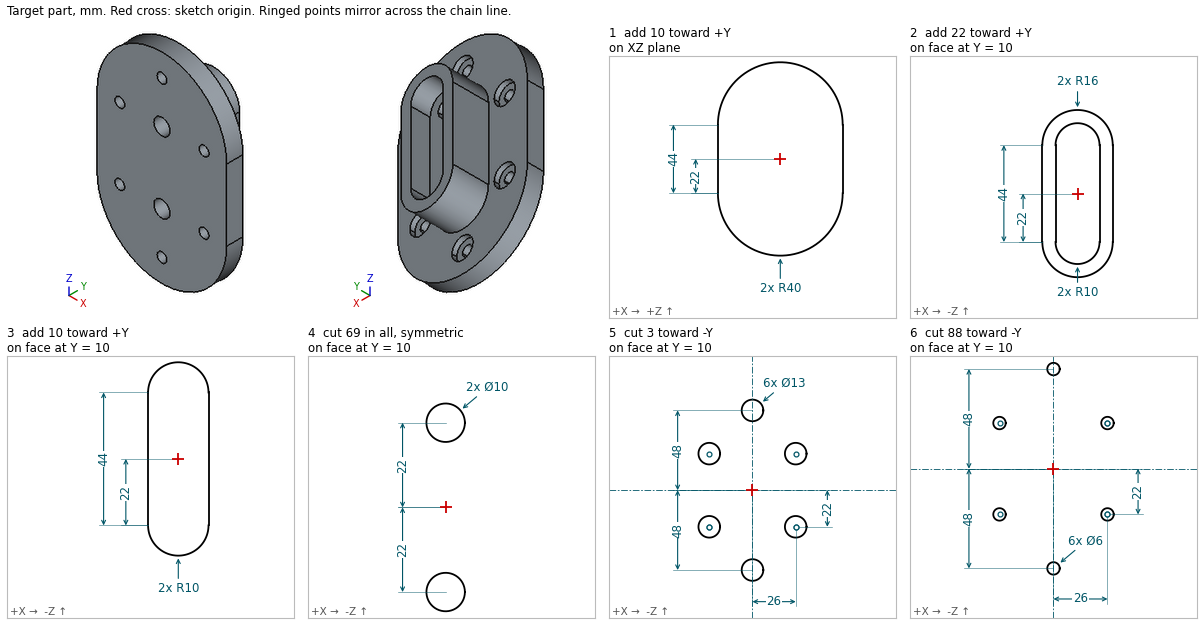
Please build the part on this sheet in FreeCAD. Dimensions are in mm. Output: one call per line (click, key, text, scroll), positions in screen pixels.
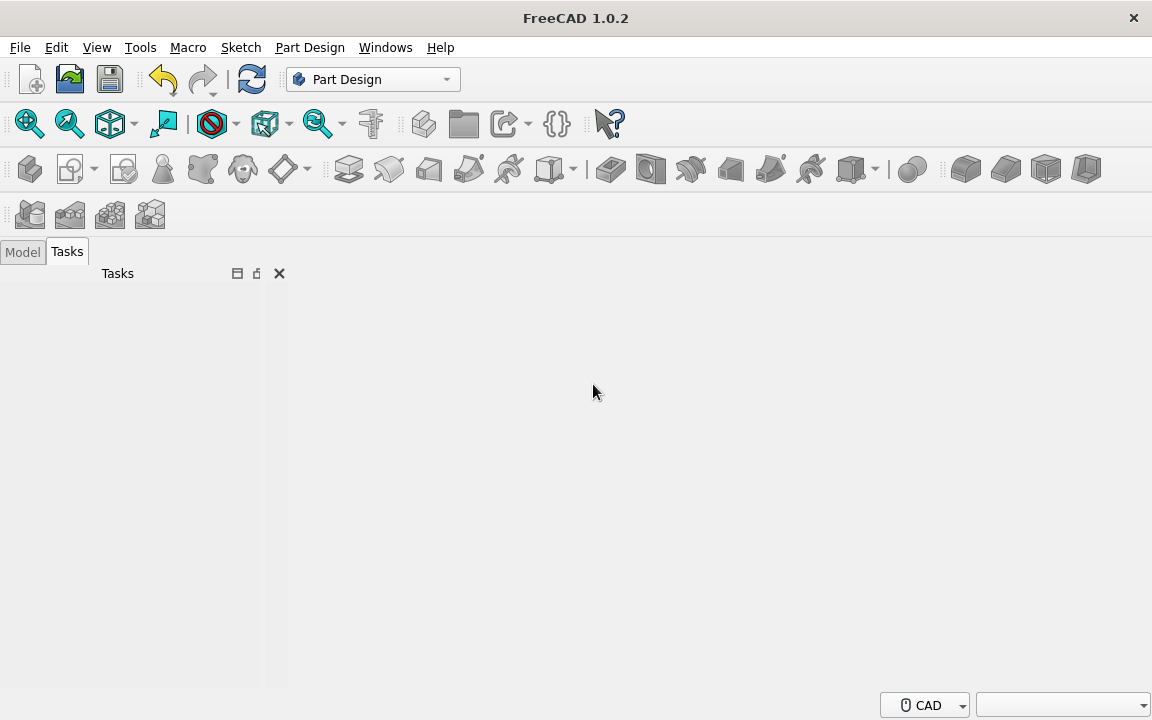
click(30, 80)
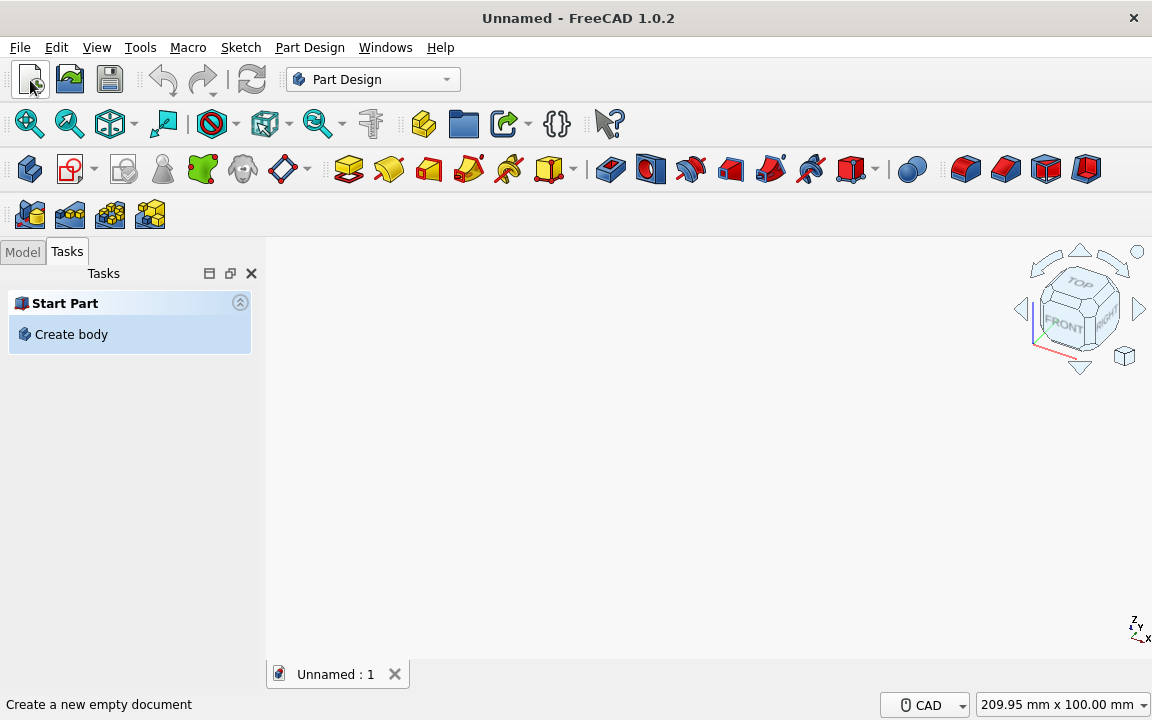
click(70, 170)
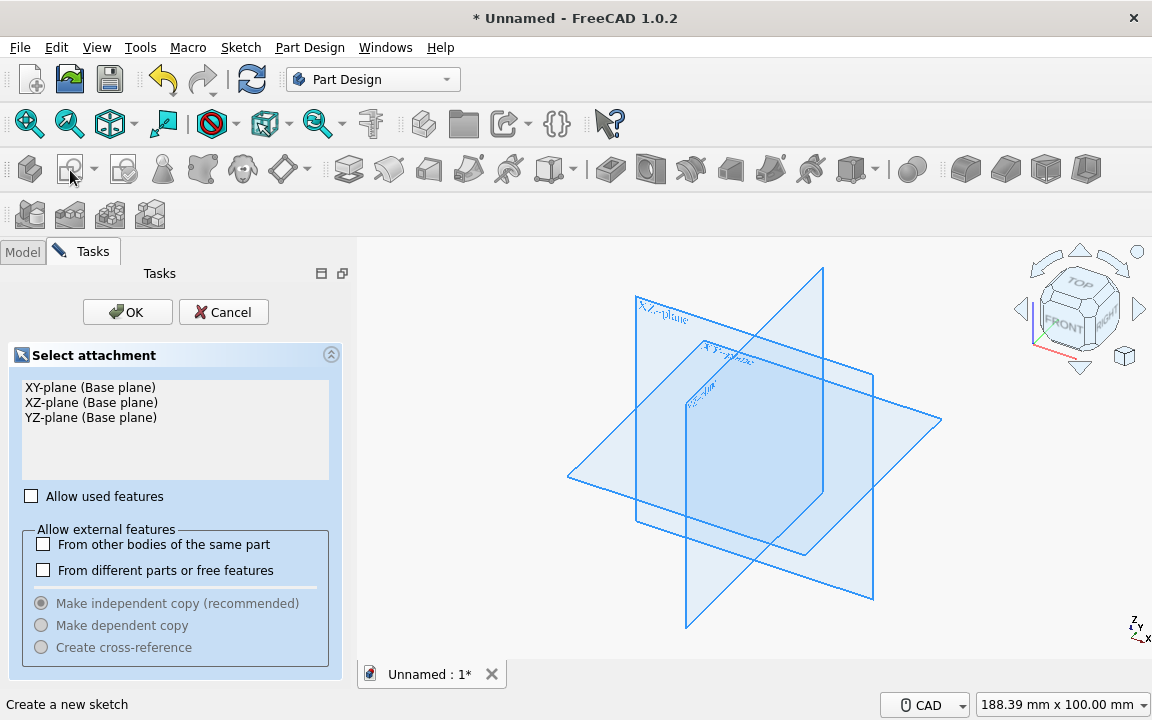
click(82, 402)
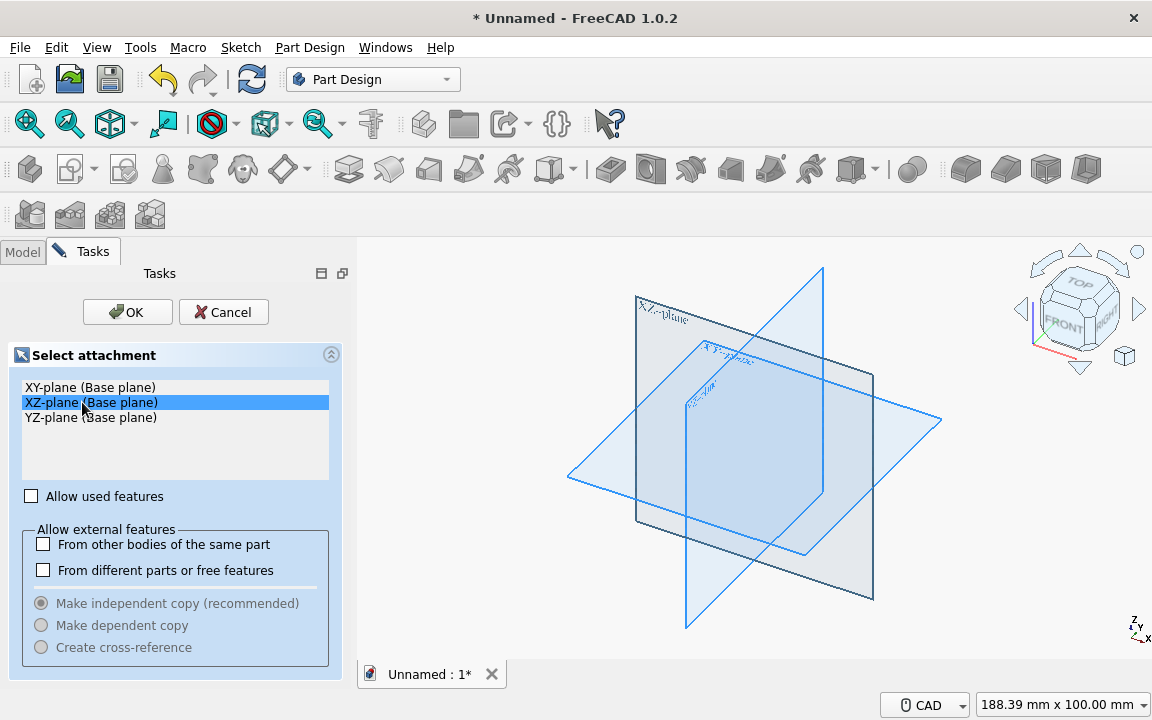
click(128, 312)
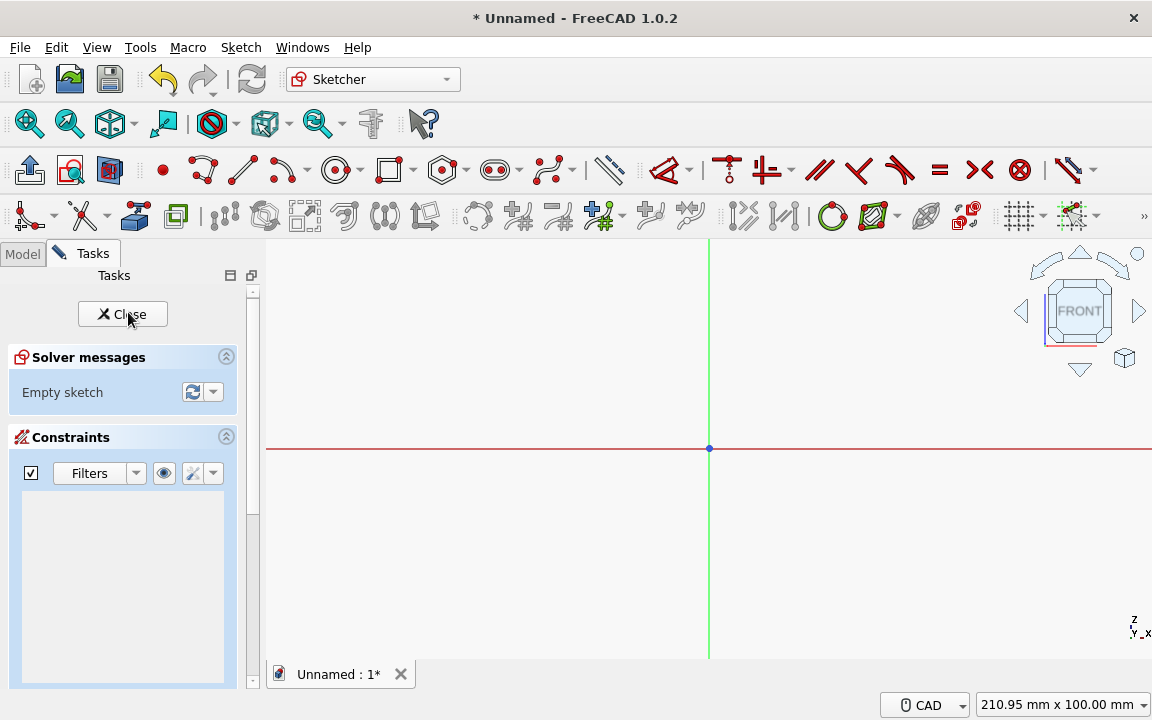
scroll(585, 449, down, 4)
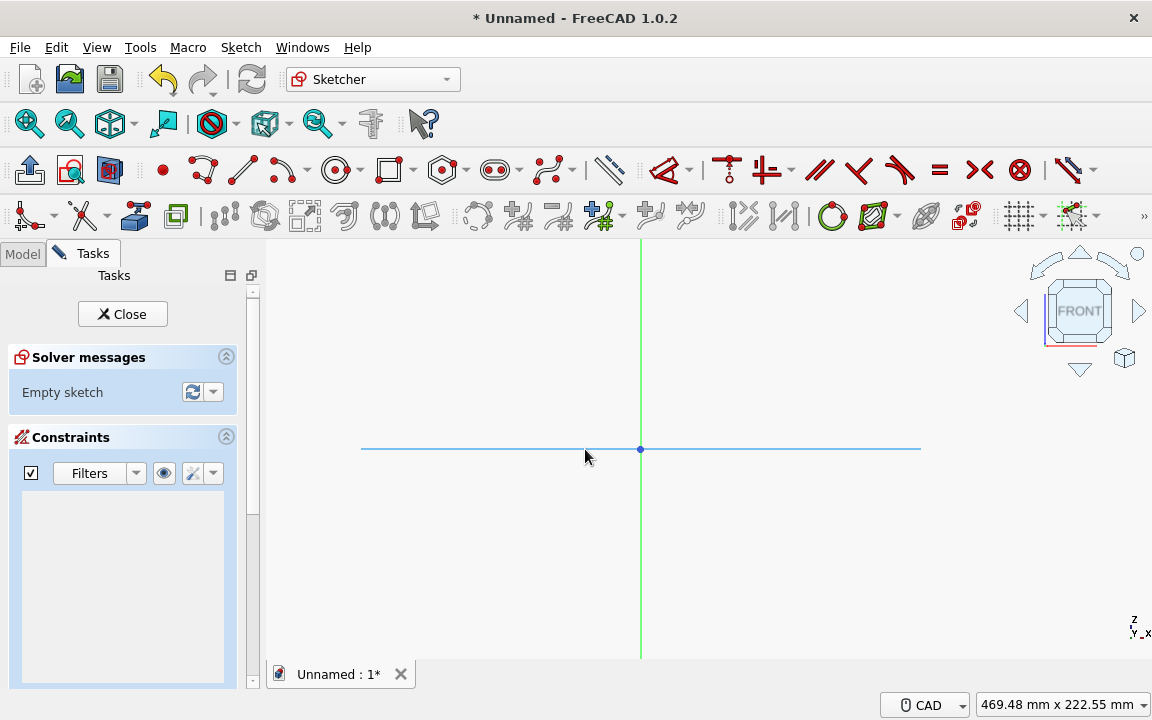
click(496, 170)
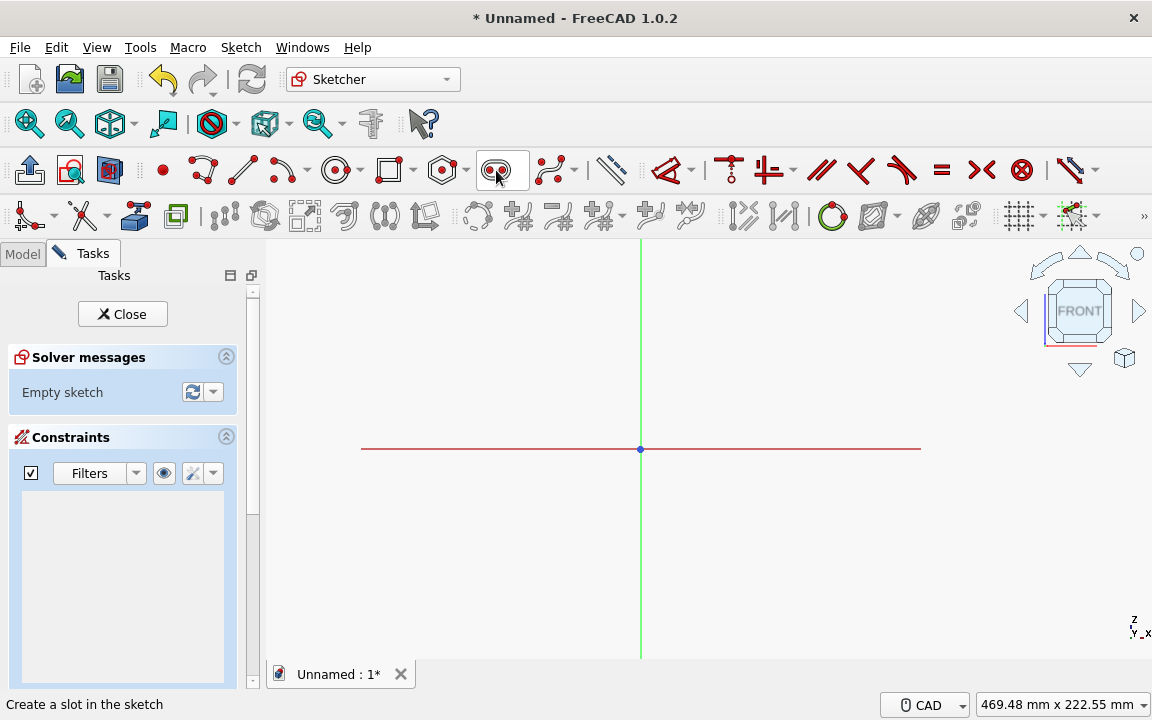
click(641, 491)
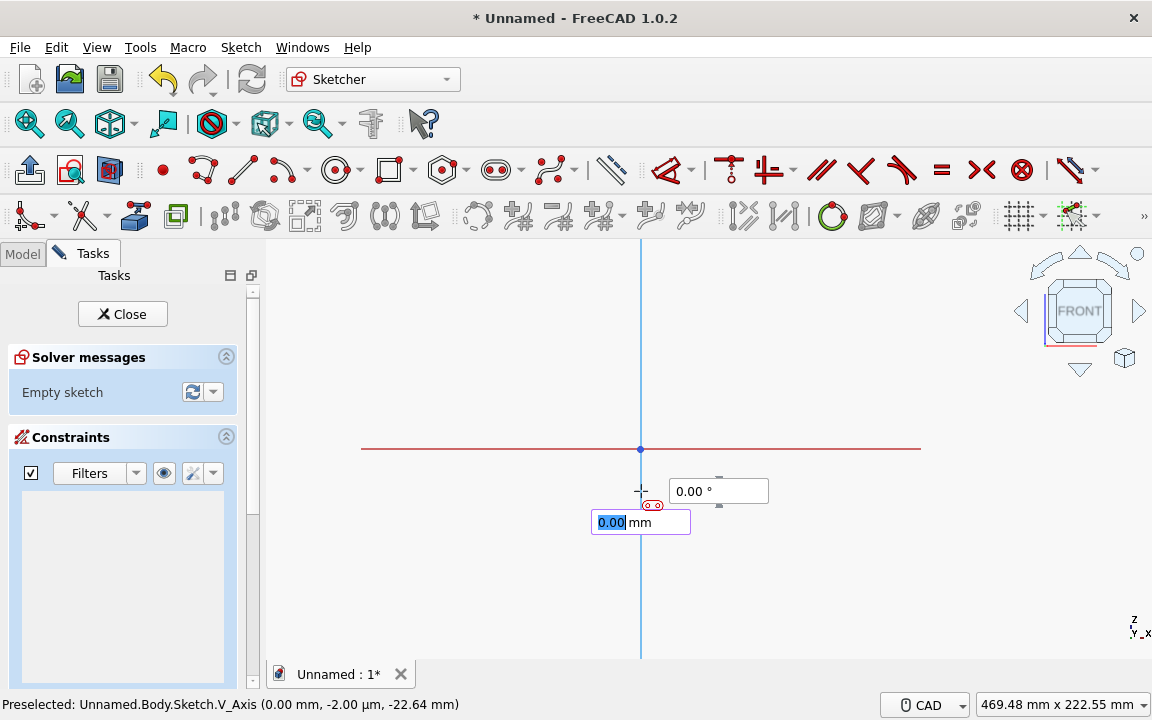
click(650, 408)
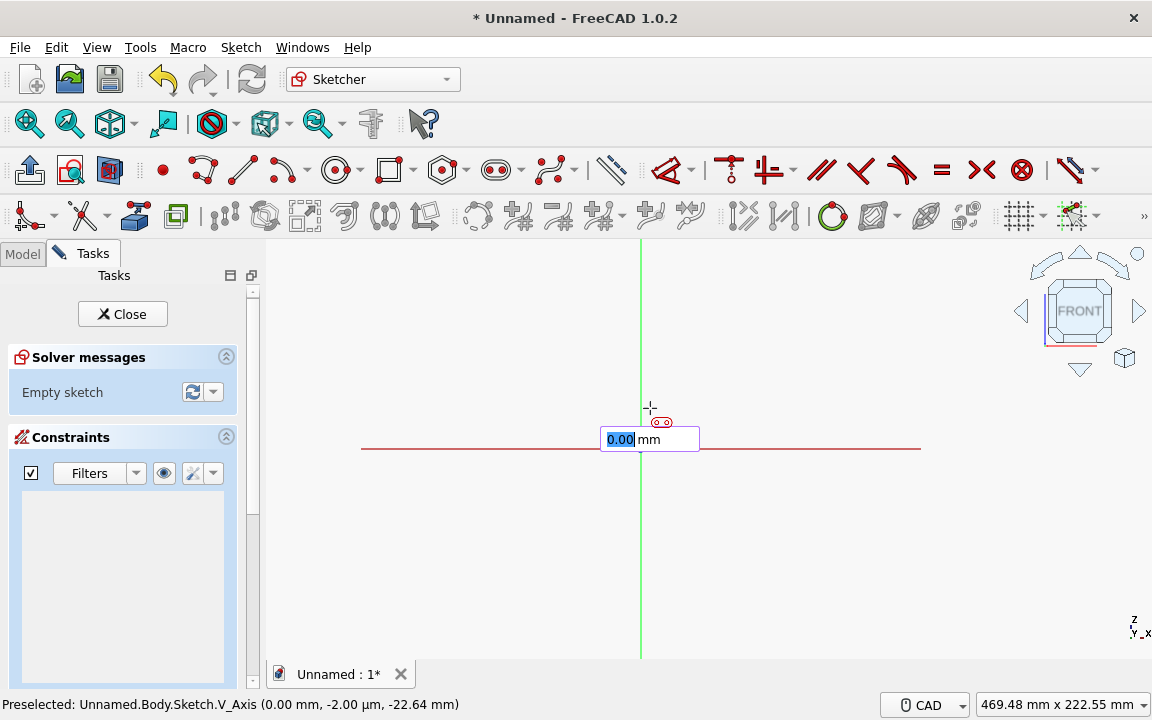
scroll(716, 437, up, 2)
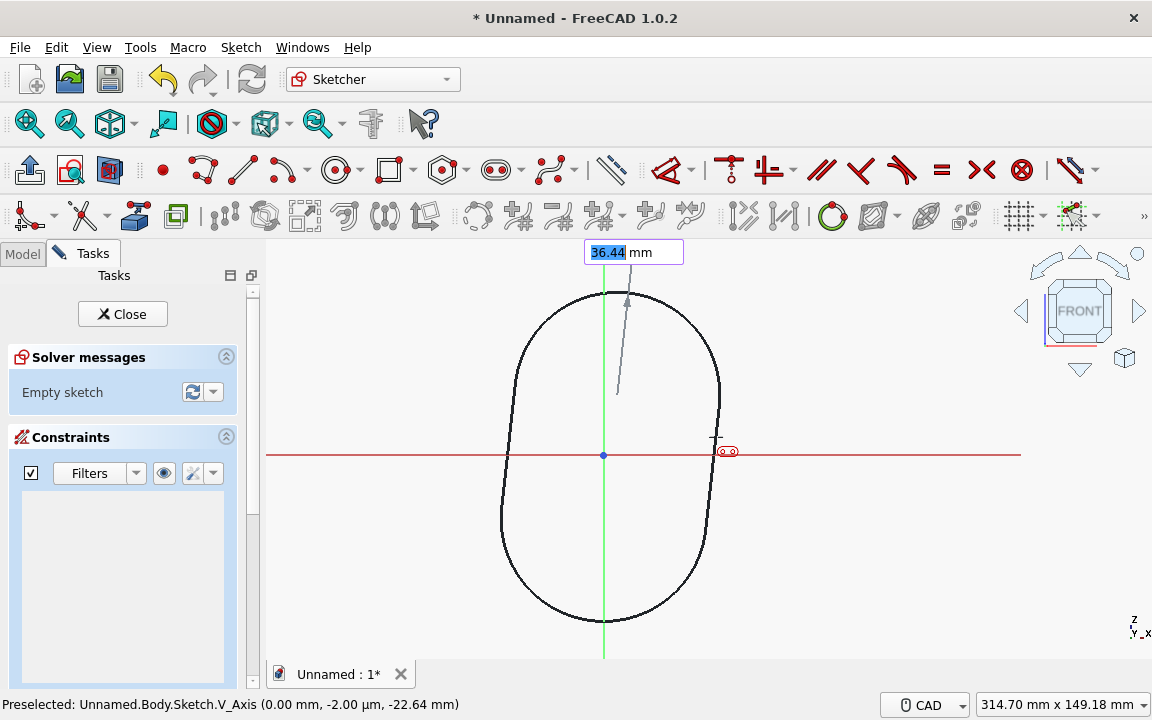
click(716, 436)
key(Escape)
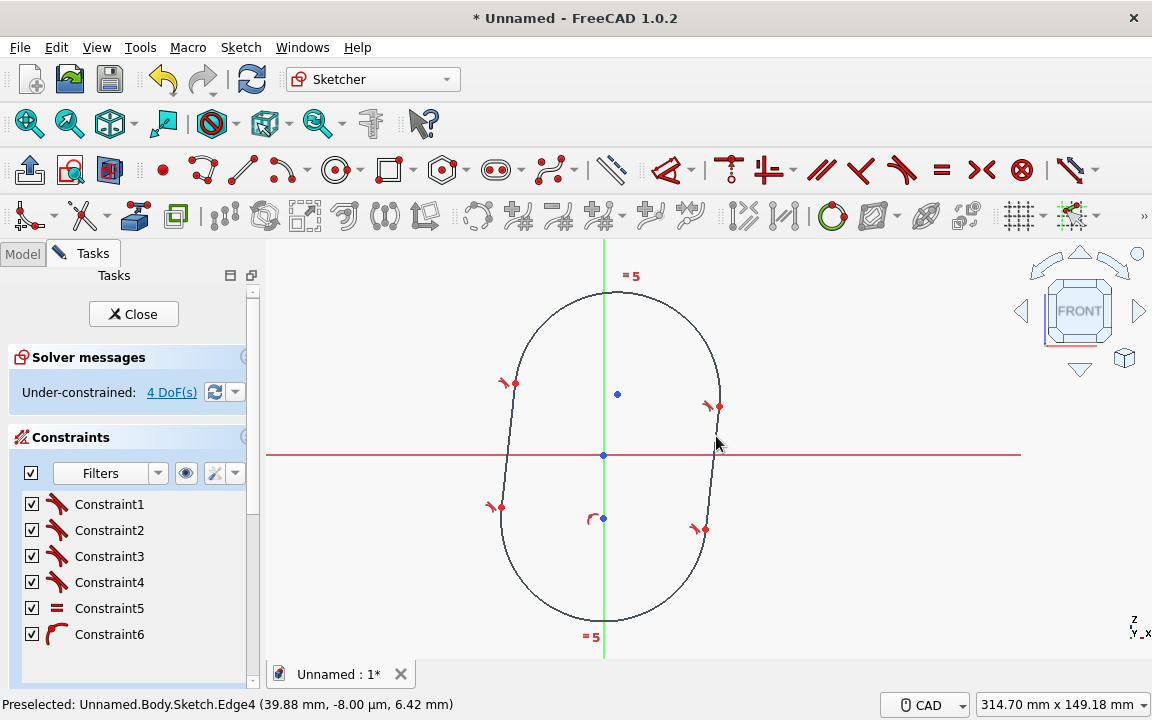
click(506, 470)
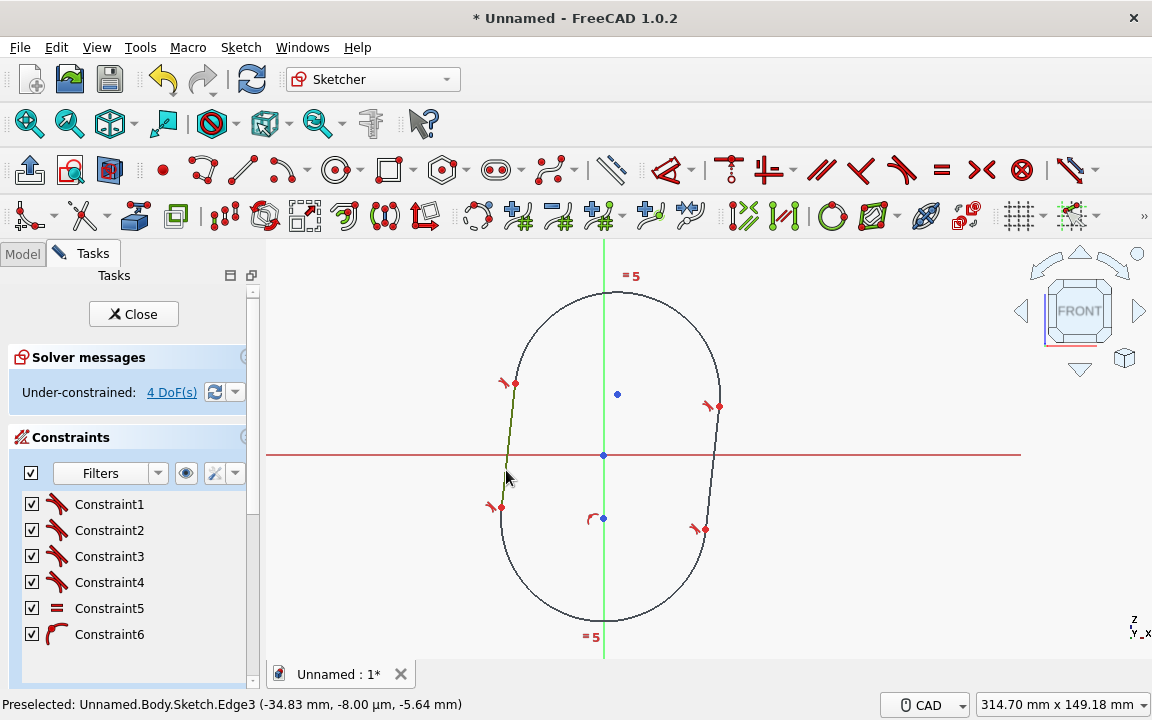
click(796, 170)